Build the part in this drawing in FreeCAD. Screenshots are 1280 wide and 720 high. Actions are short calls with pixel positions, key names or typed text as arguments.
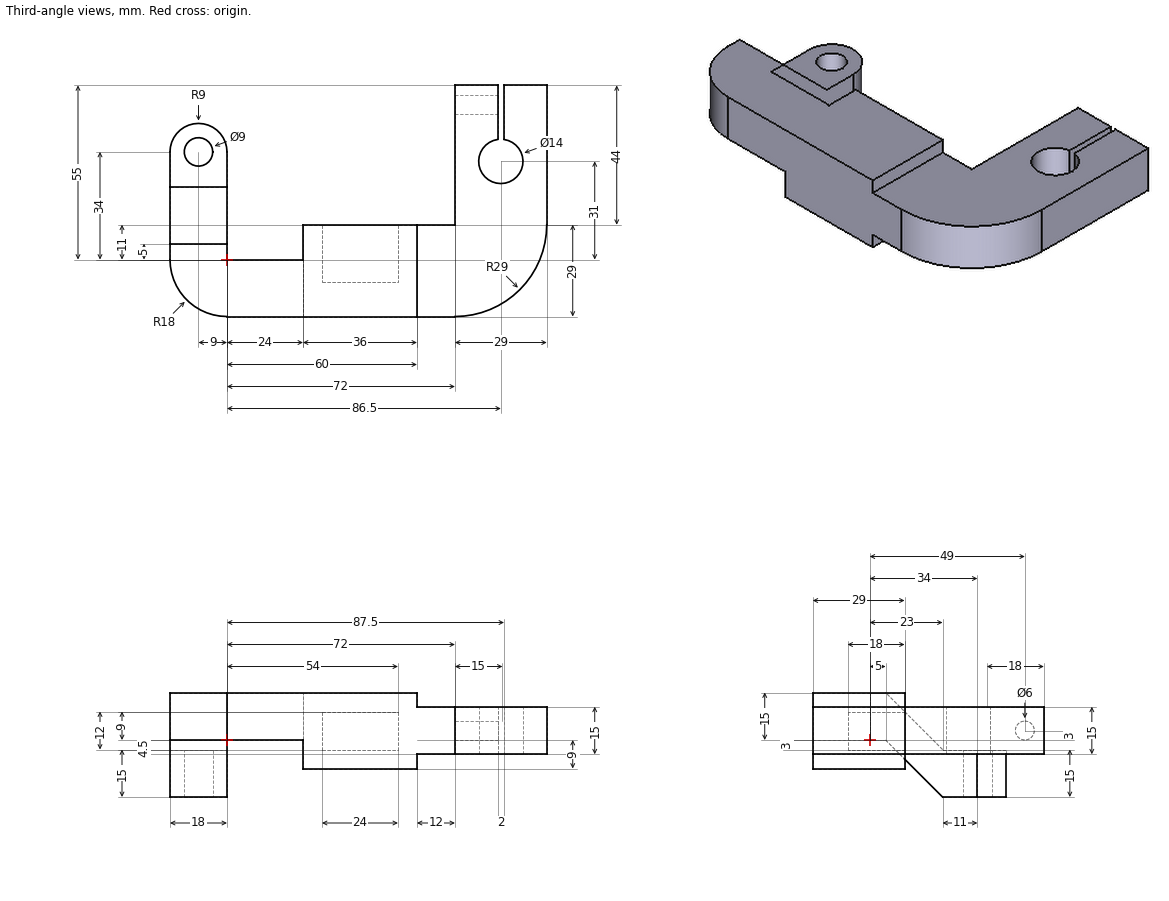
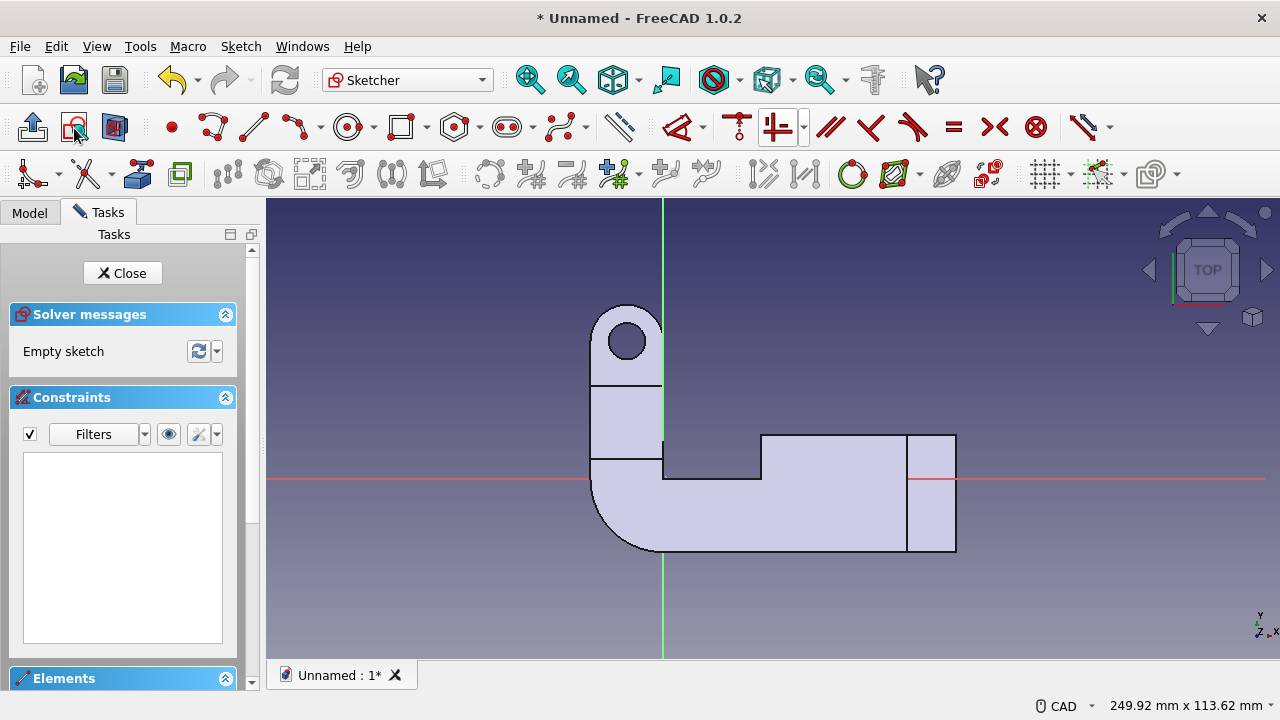
click(115, 128)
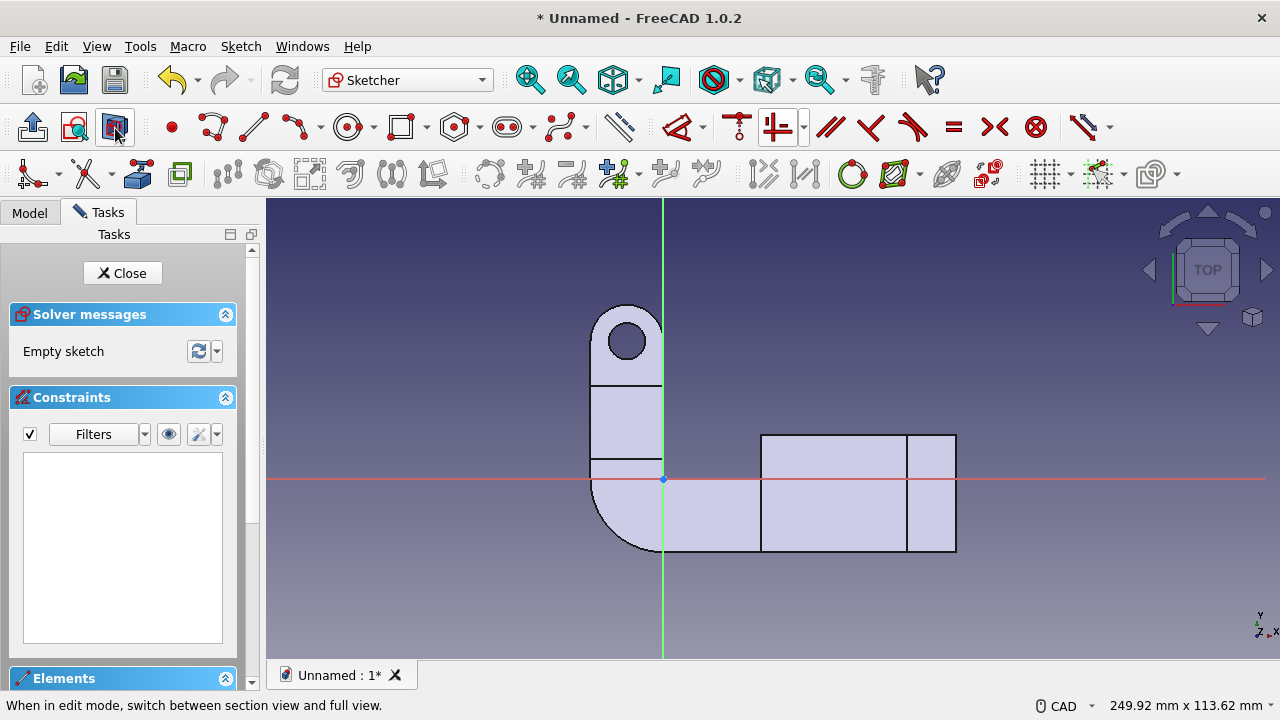
scroll(1115, 546, up, 4)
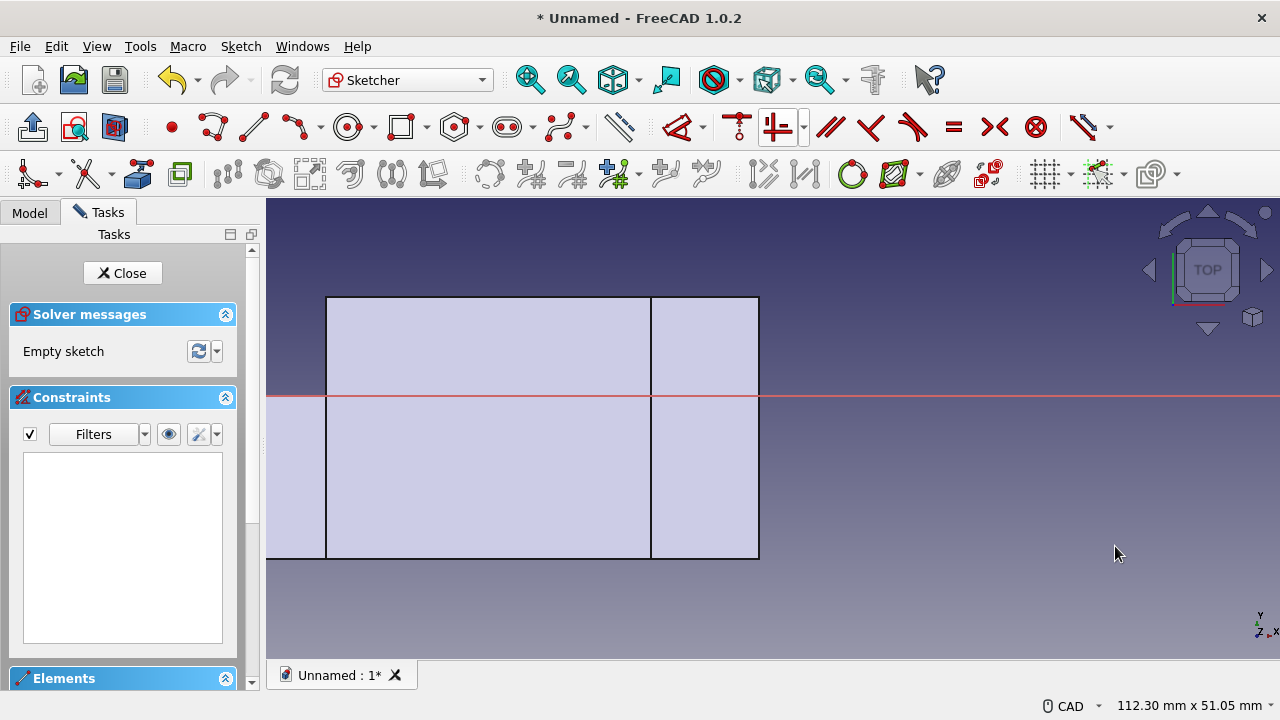
click(213, 128)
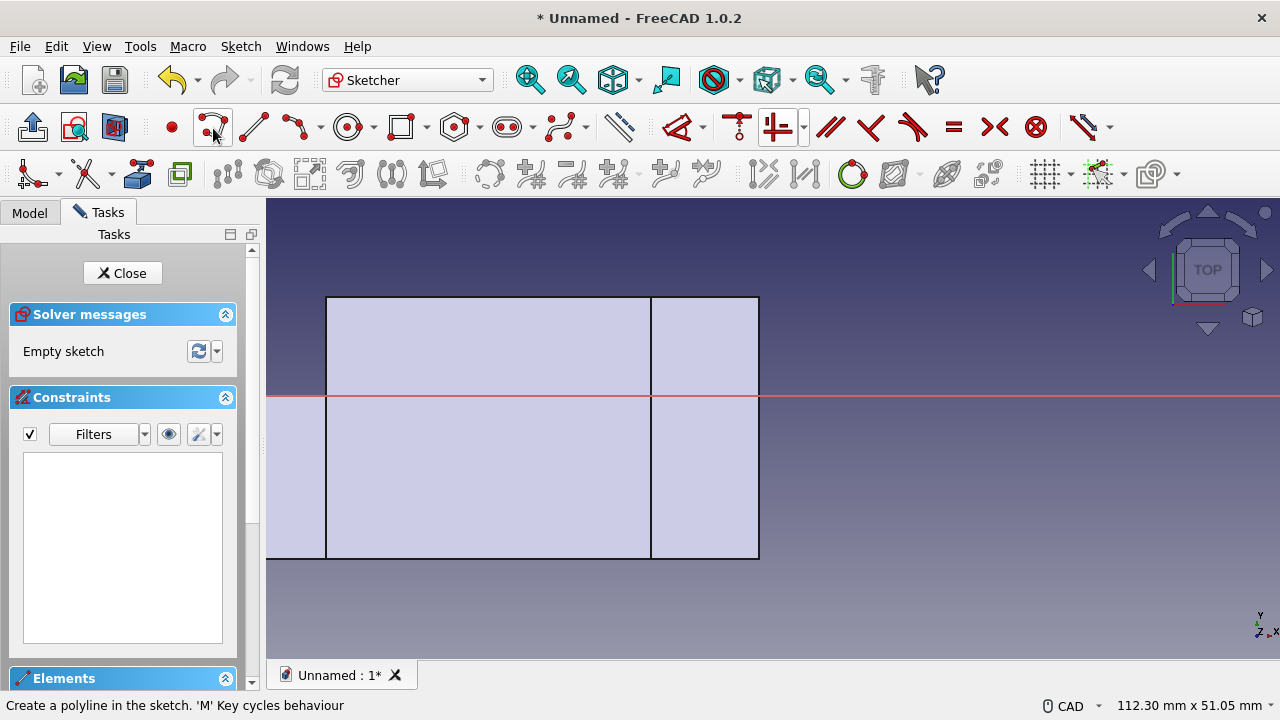
click(1021, 297)
click(759, 297)
click(759, 559)
right_click(759, 559)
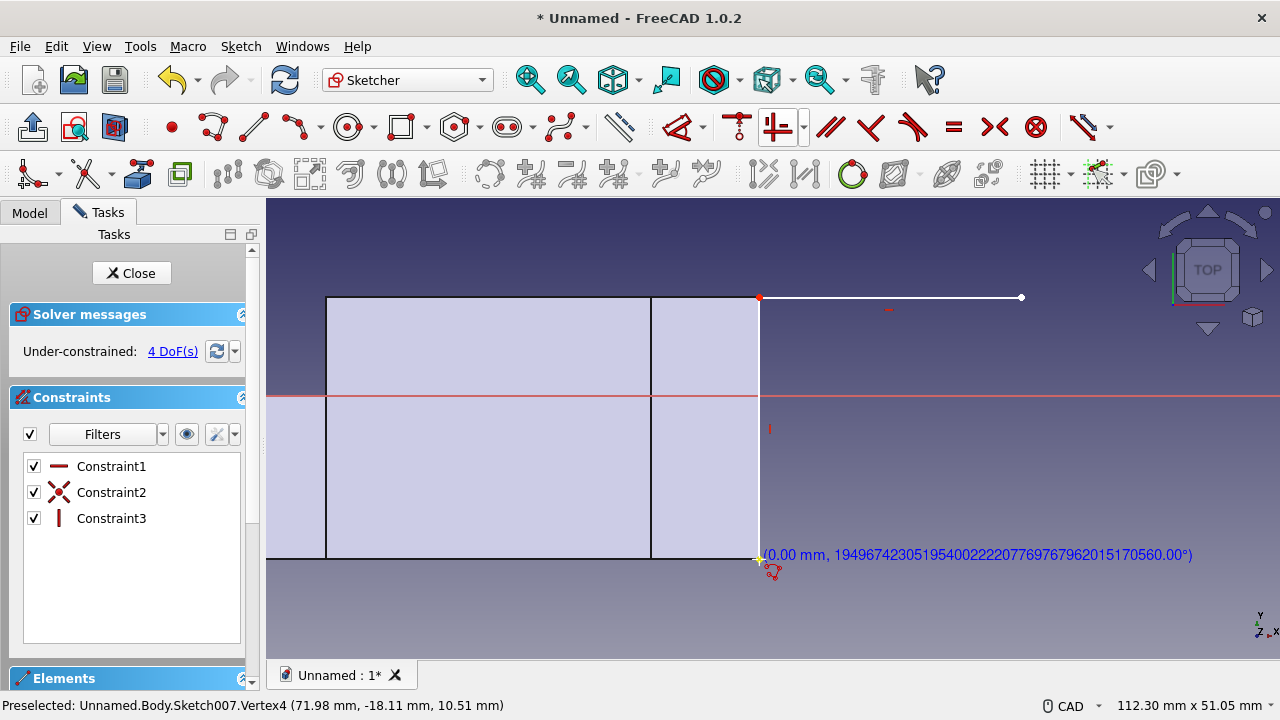
click(294, 128)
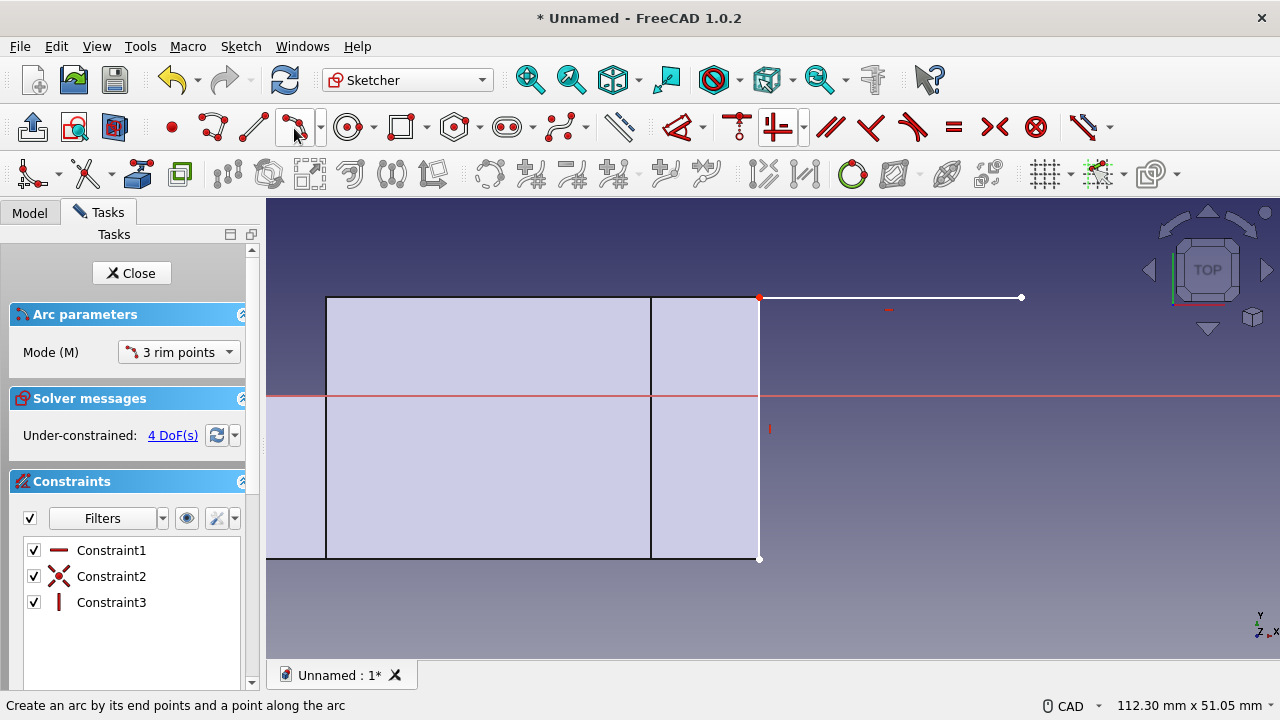
click(759, 560)
click(1021, 298)
click(944, 482)
key(Escape)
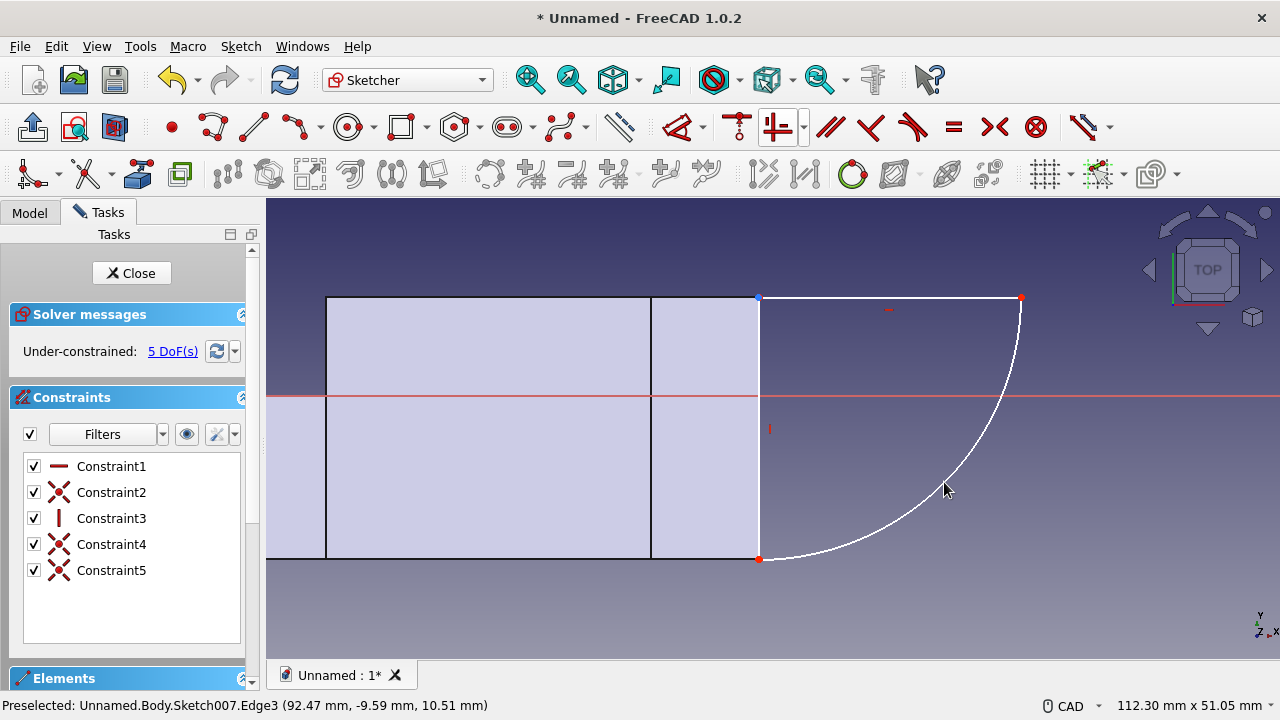
click(676, 128)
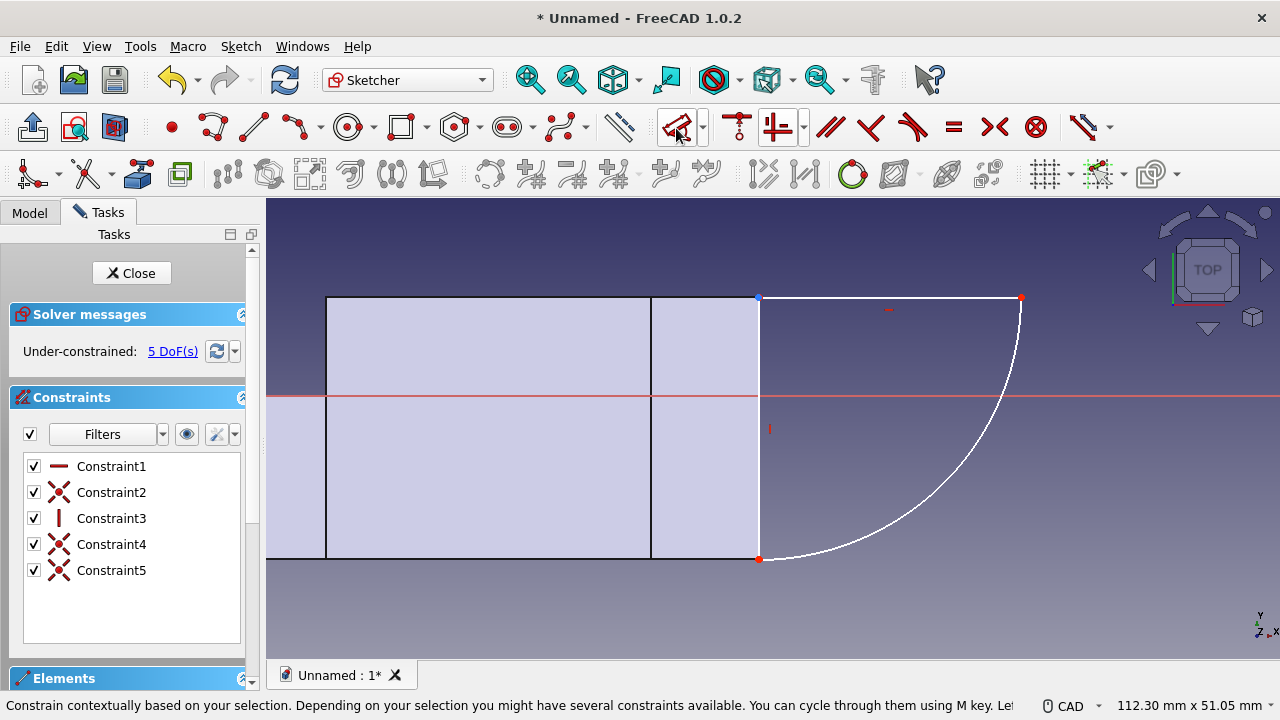
click(878, 531)
click(893, 559)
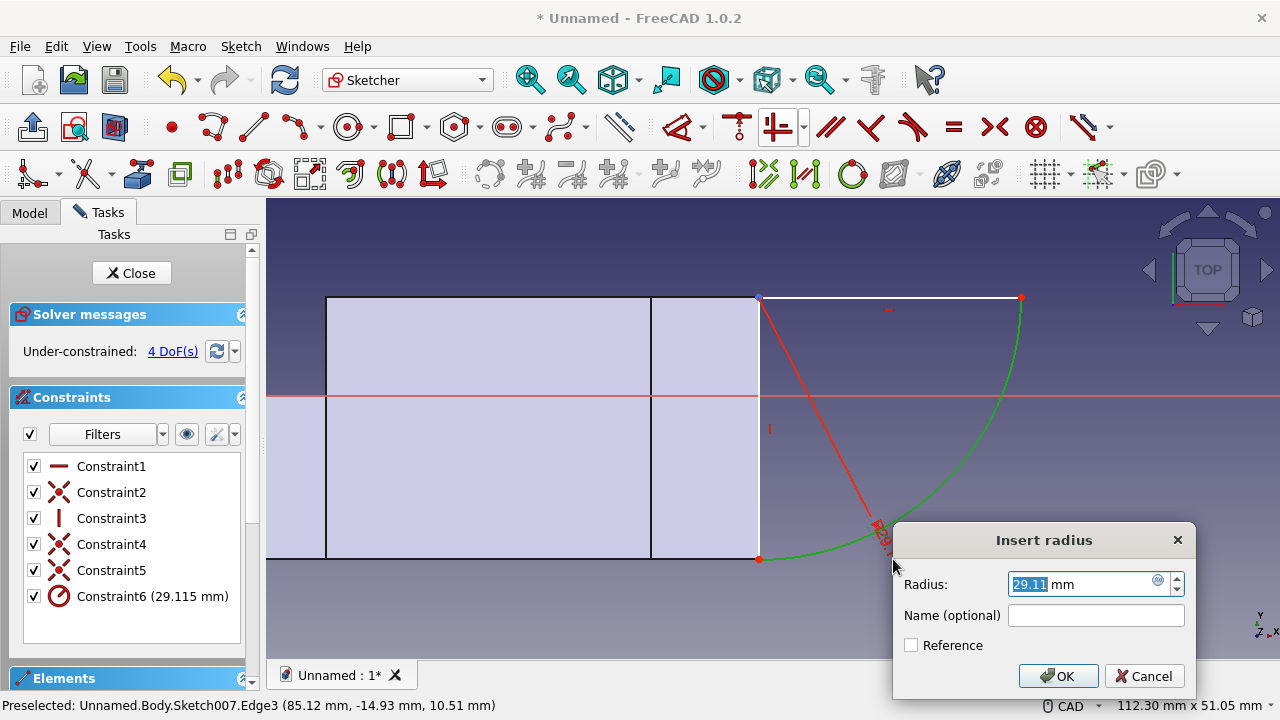
text(29)
key(Return)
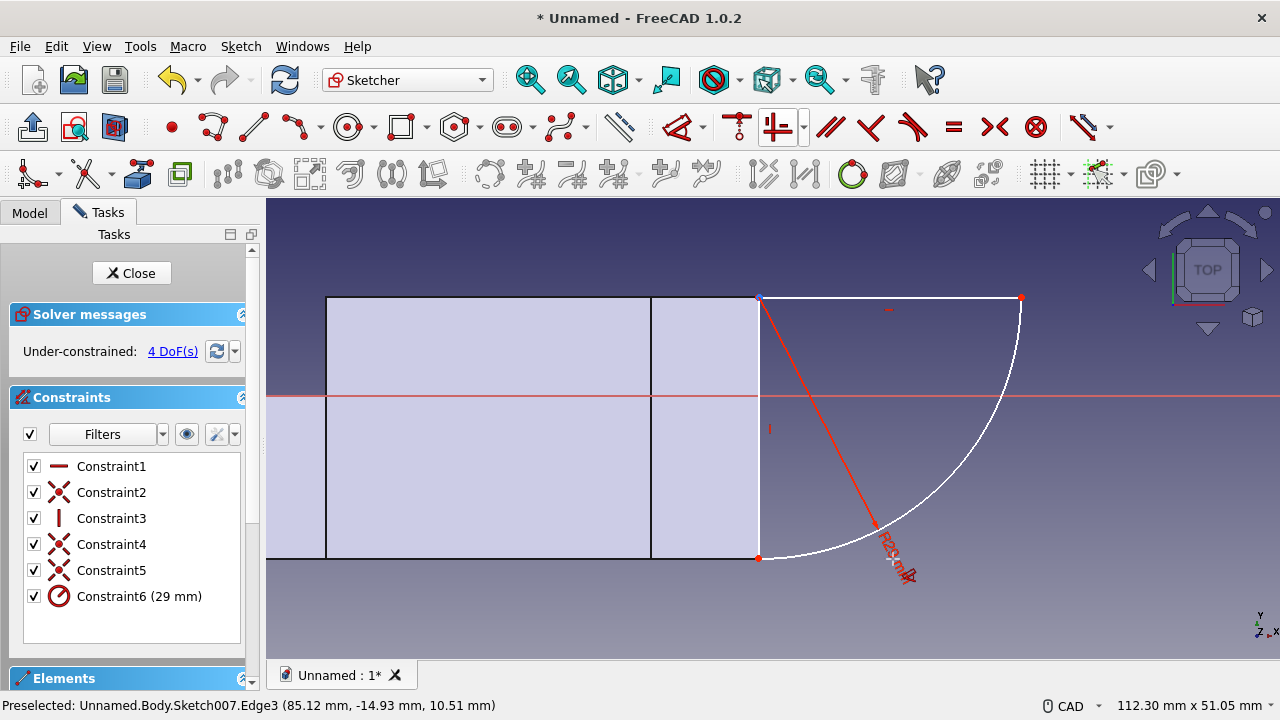
click(942, 298)
click(890, 264)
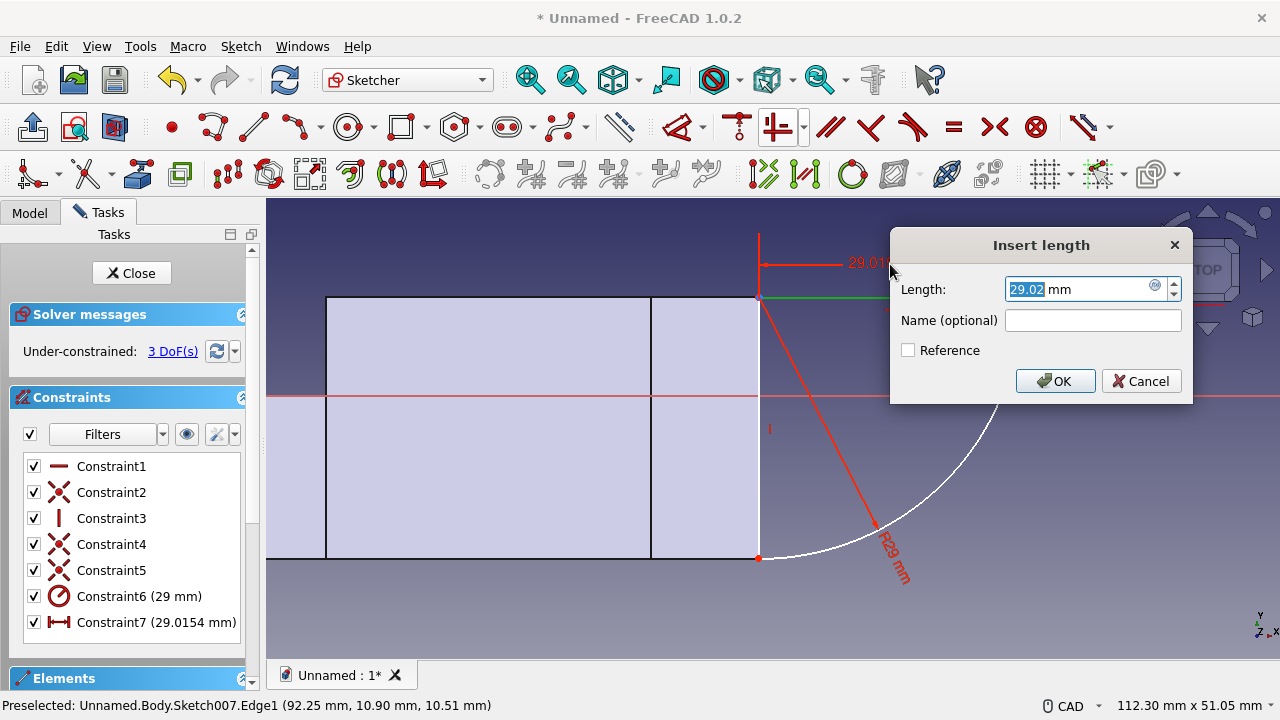
text(29)
key(Return)